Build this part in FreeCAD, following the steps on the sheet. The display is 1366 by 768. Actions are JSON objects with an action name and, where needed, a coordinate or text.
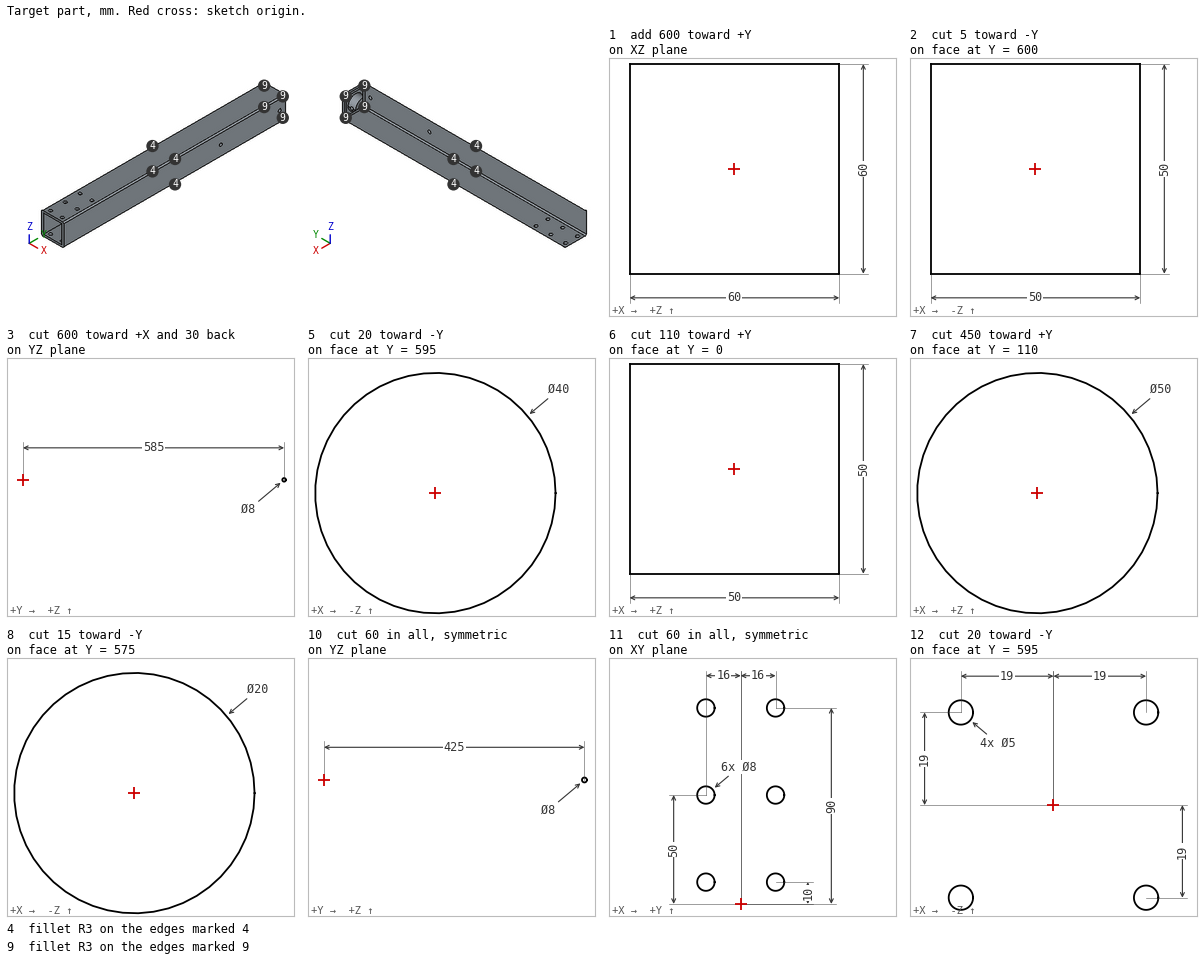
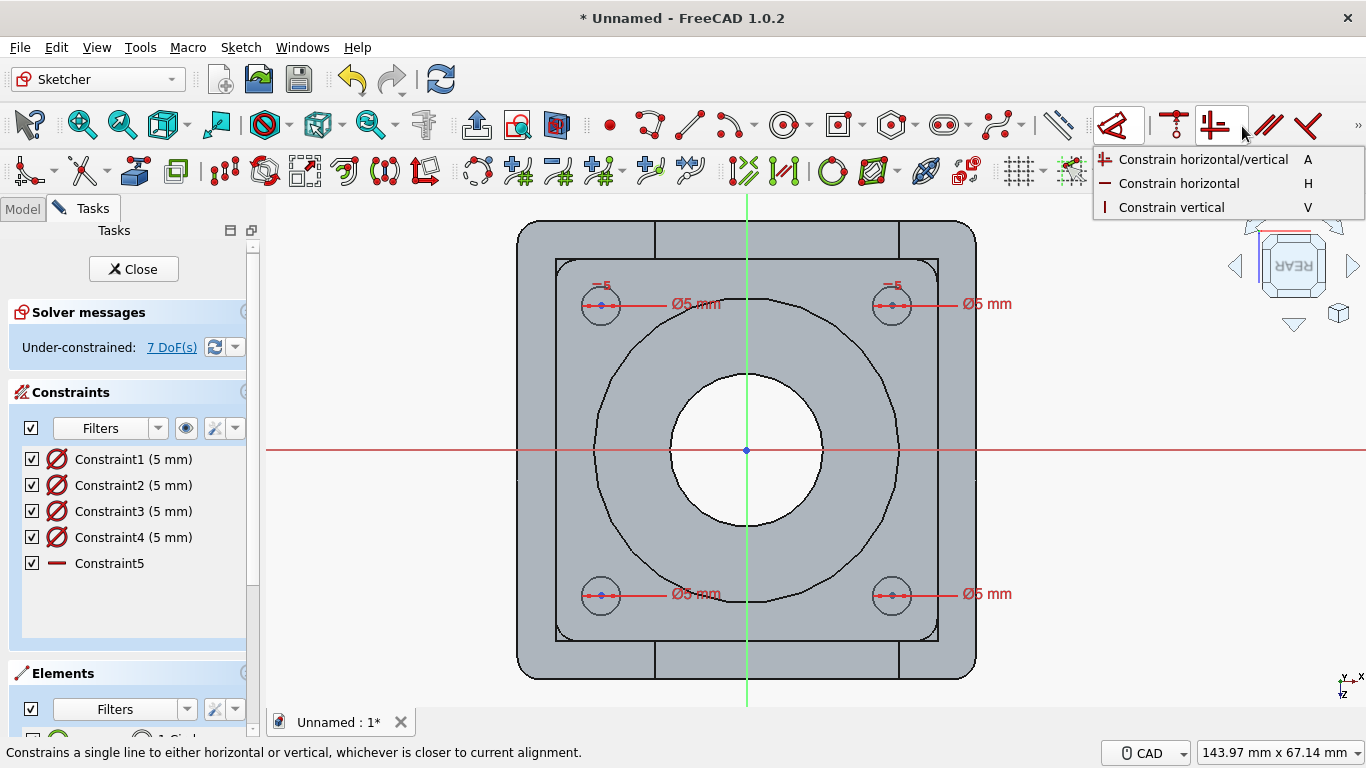
{"action": "left_click", "coordinate": [1229, 207]}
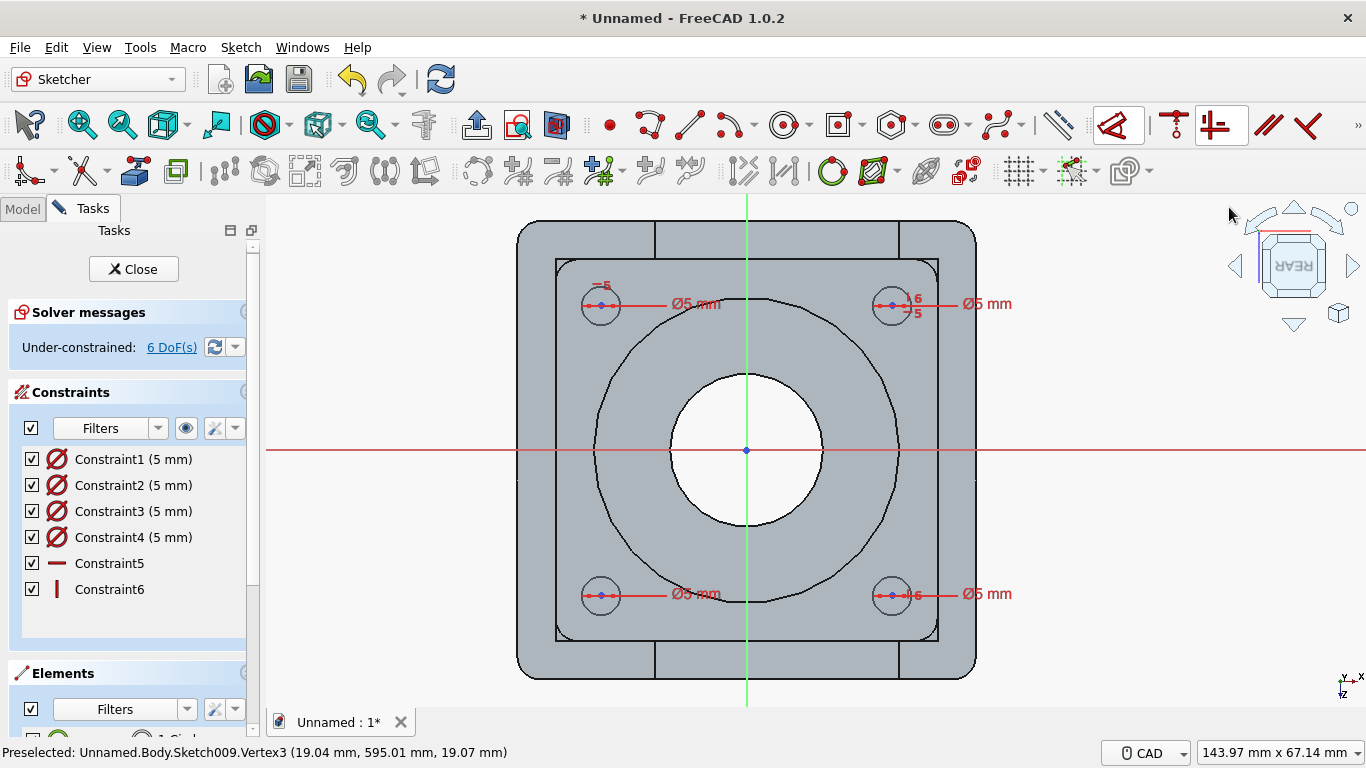
{"action": "left_click", "coordinate": [601, 306]}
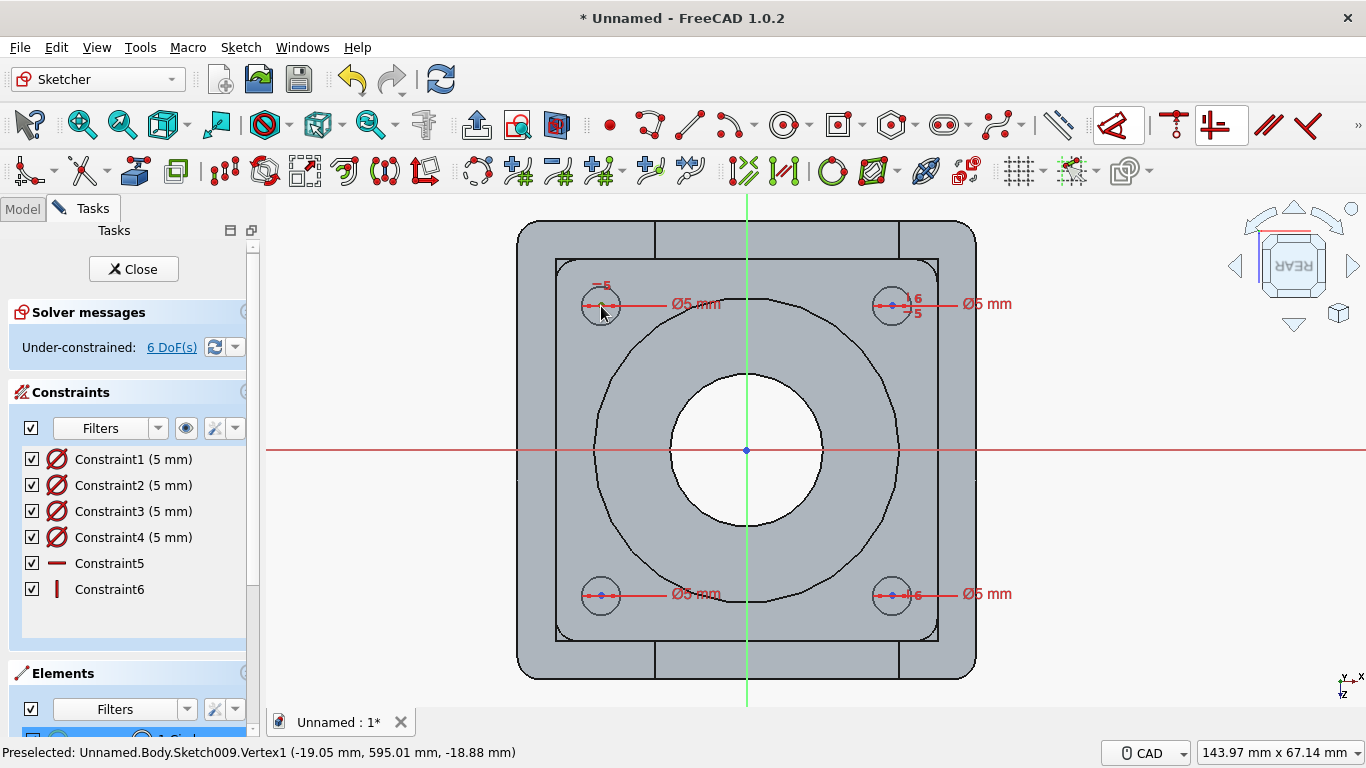
{"action": "left_click", "coordinate": [601, 596]}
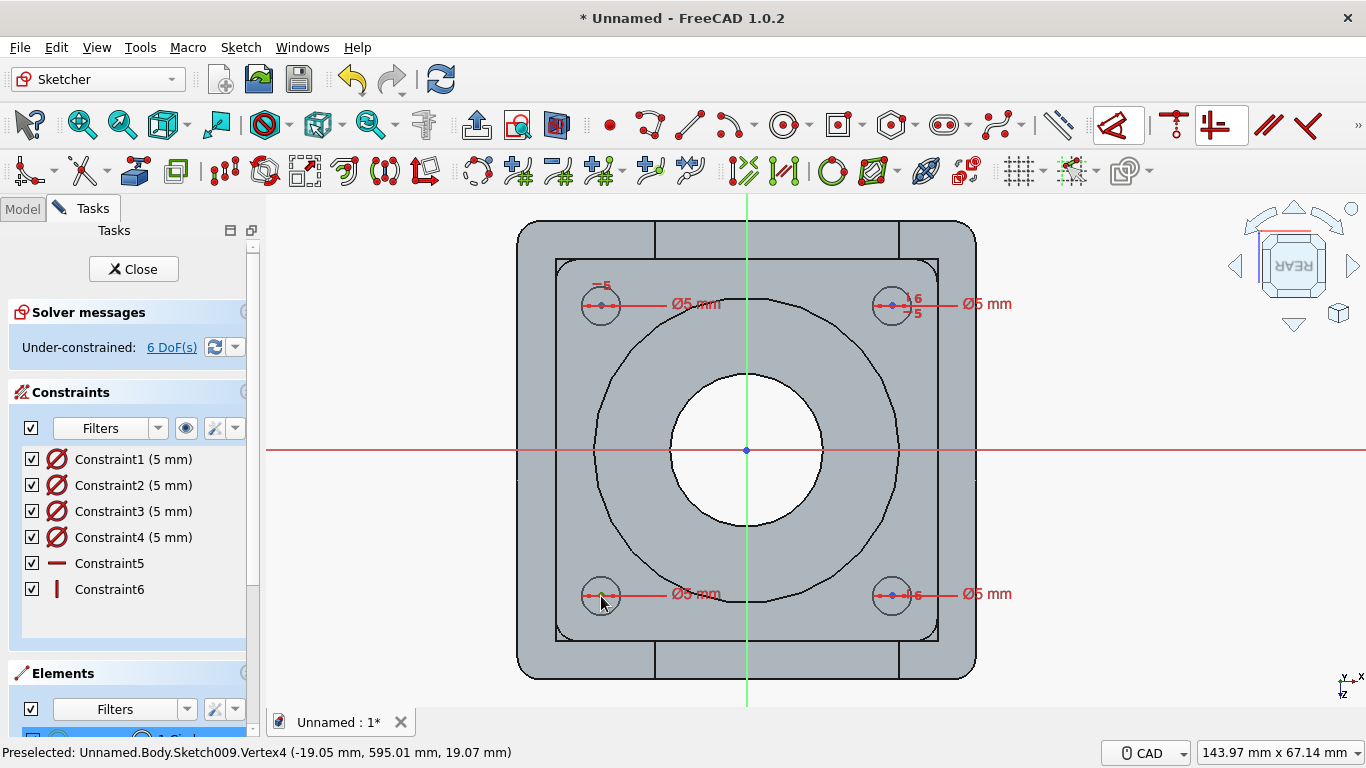
{"action": "left_click", "coordinate": [1242, 126]}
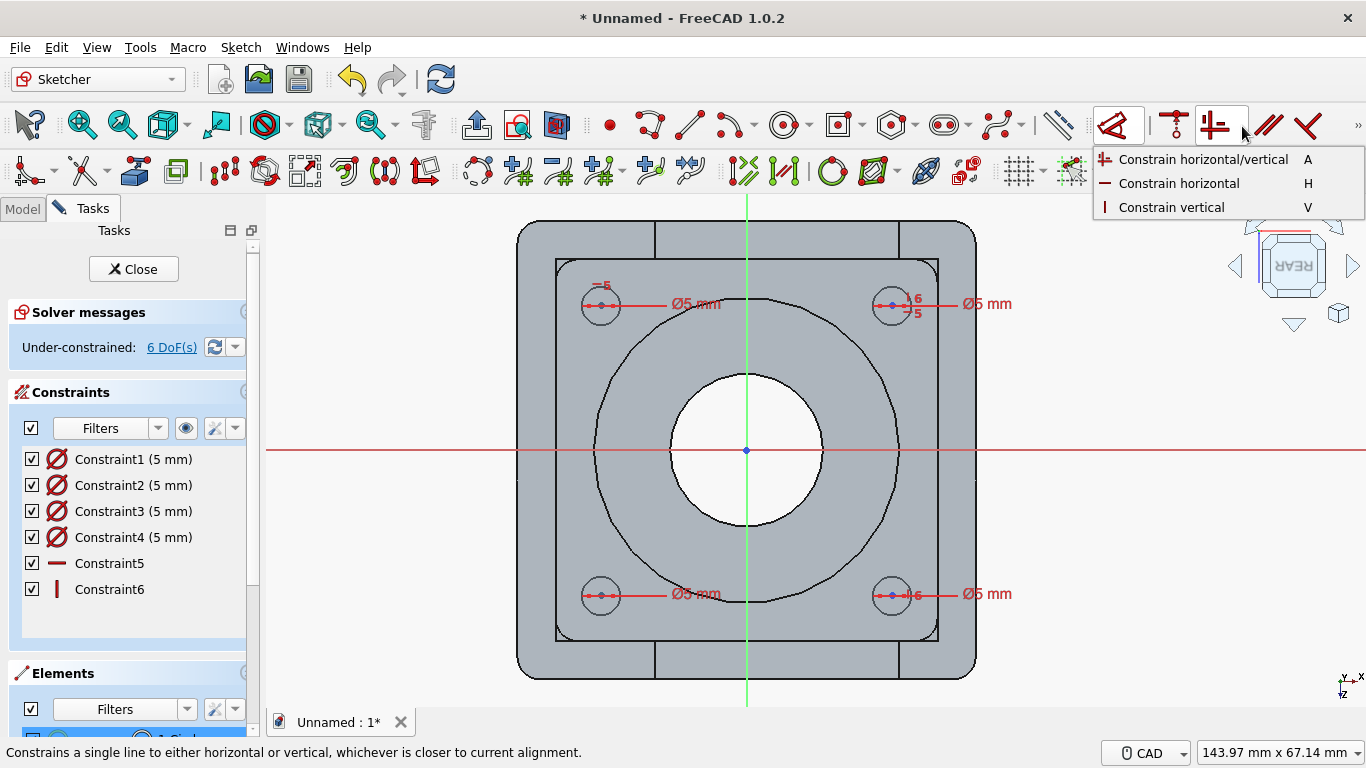
{"action": "left_click", "coordinate": [1229, 207]}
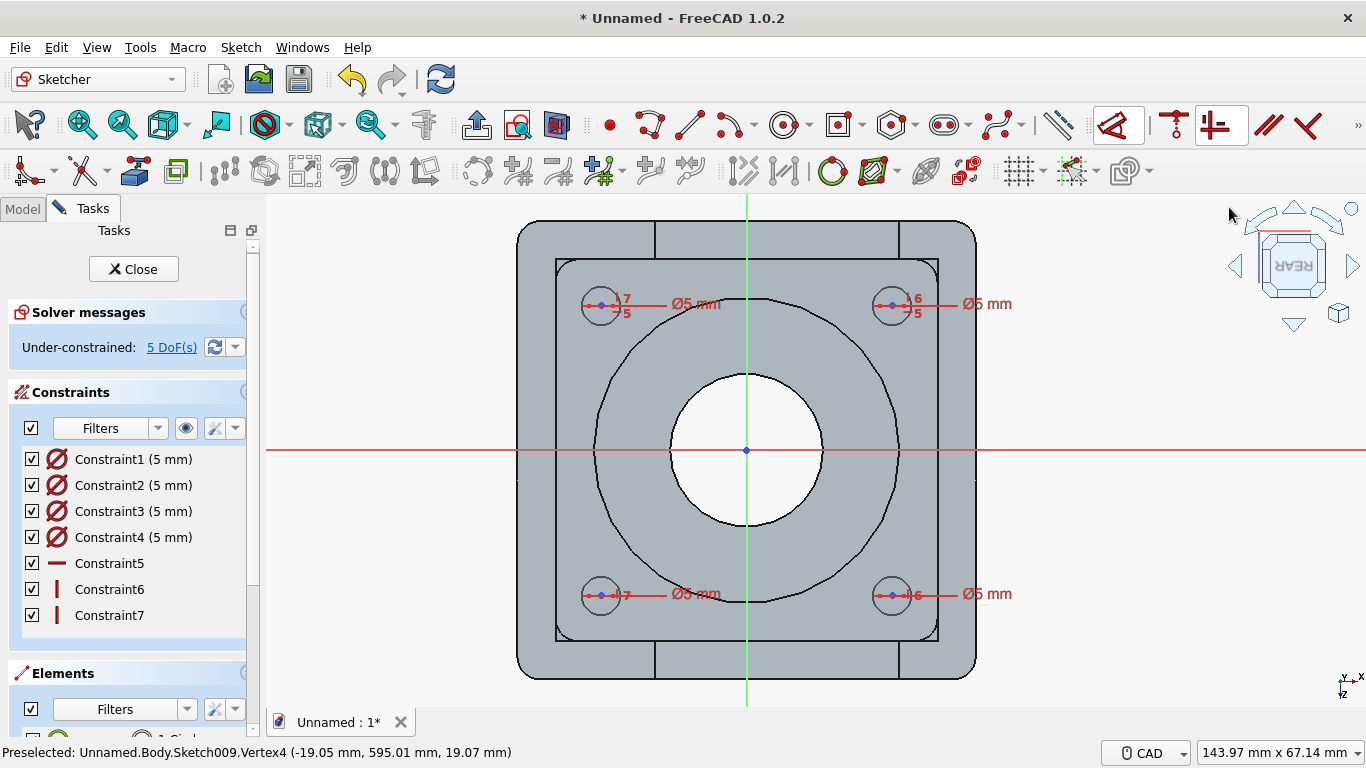
{"action": "left_click", "coordinate": [892, 596]}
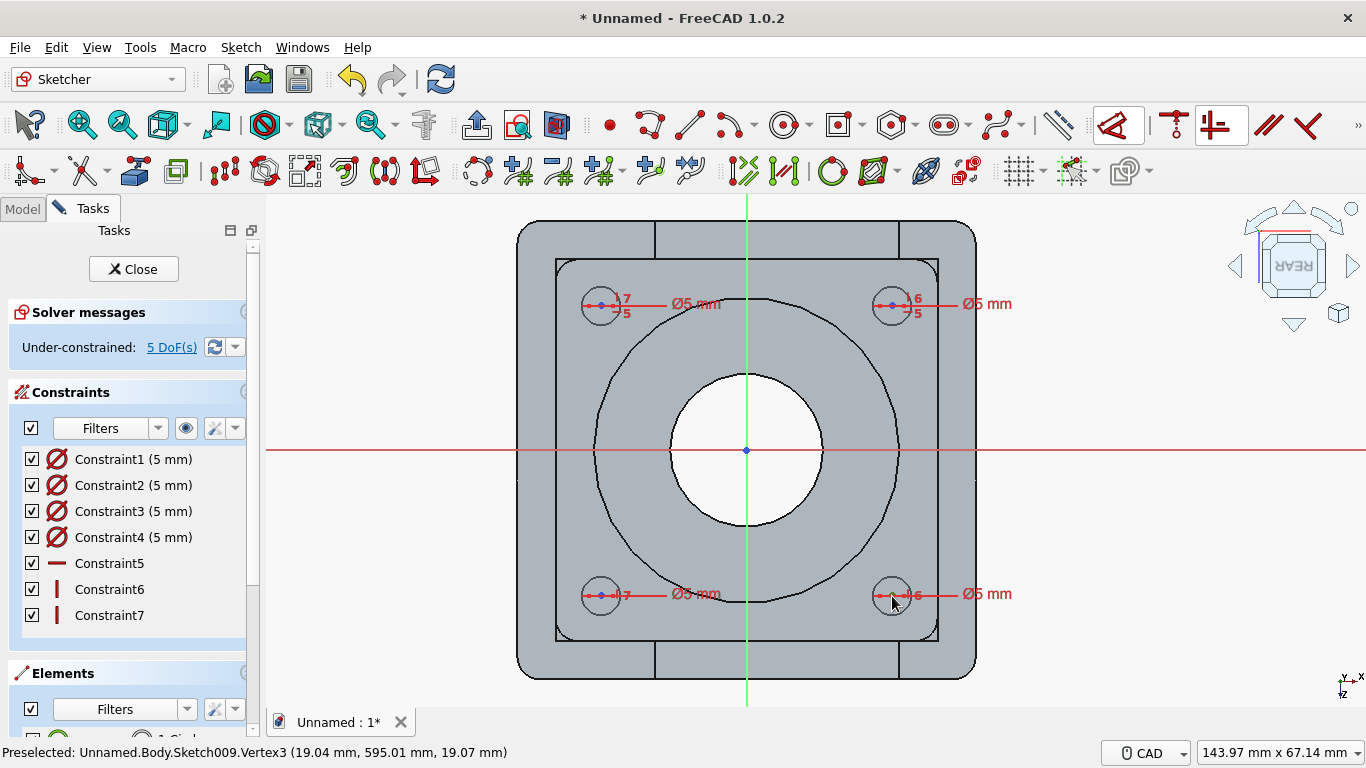
{"action": "left_click", "coordinate": [601, 596]}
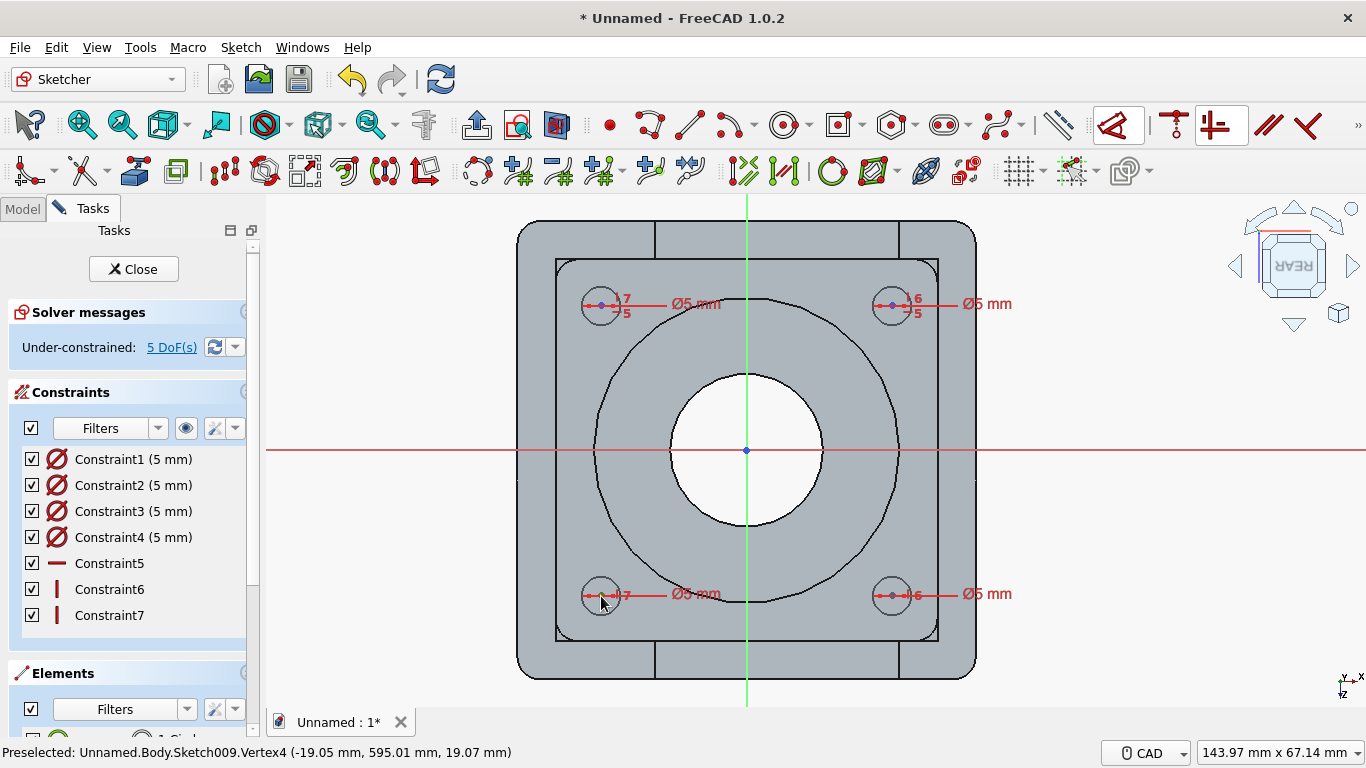
{"action": "key", "text": "h"}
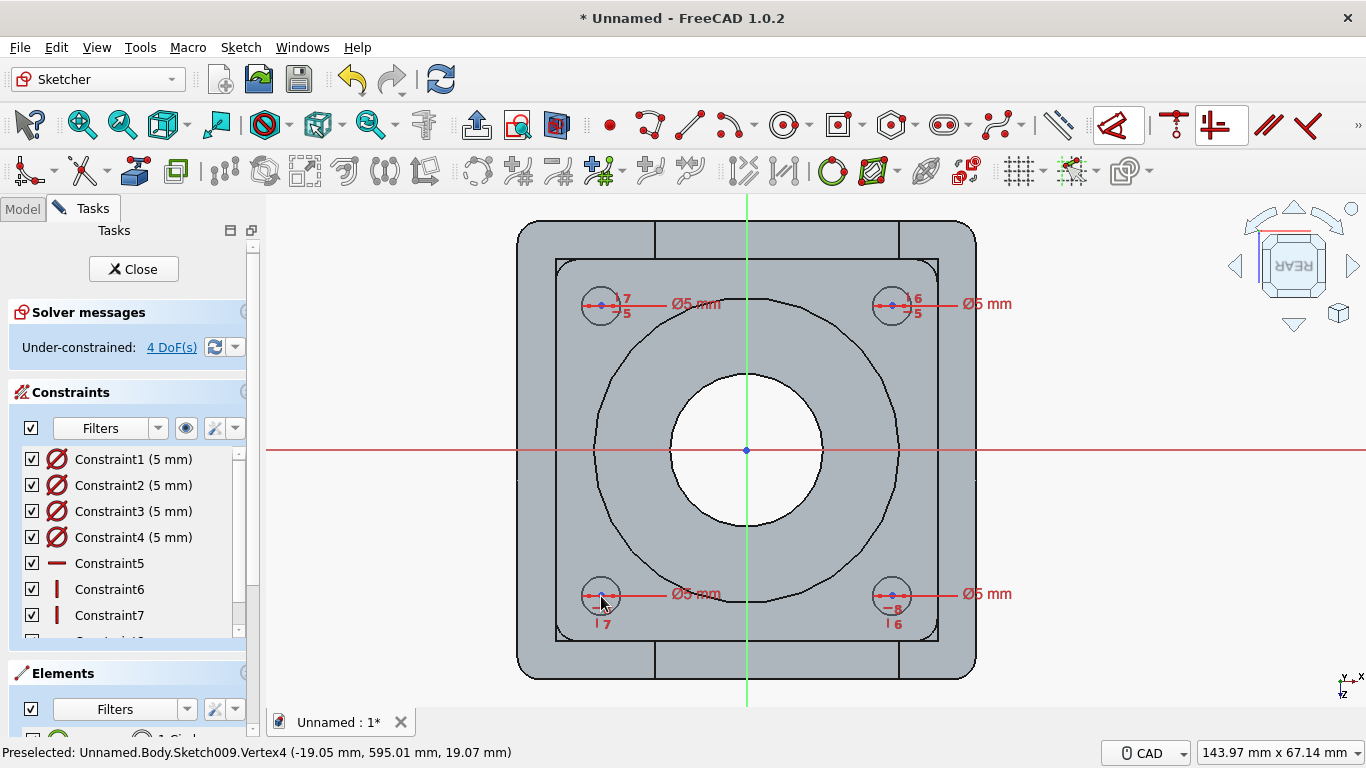
{"action": "left_click", "coordinate": [601, 306]}